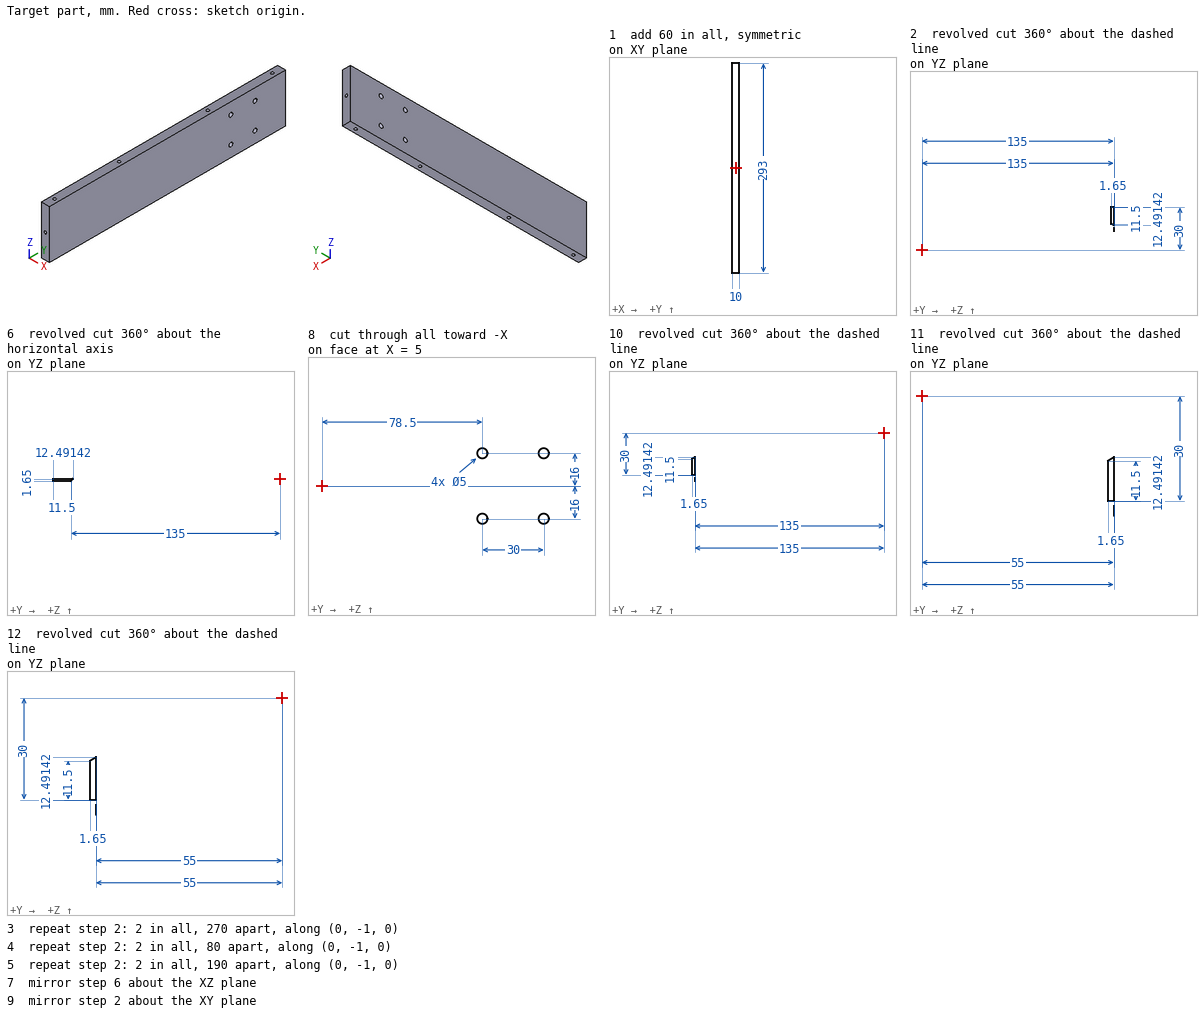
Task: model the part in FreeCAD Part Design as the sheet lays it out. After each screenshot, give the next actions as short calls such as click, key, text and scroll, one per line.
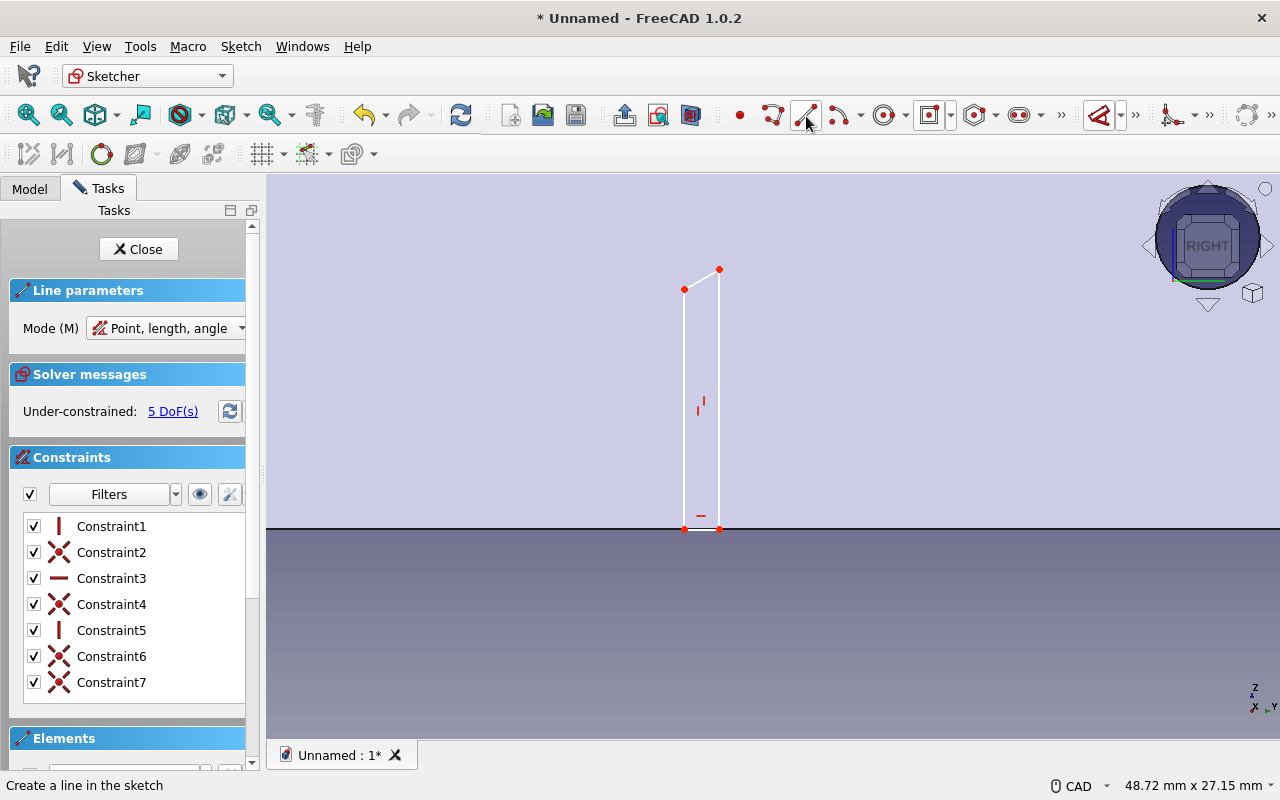
click(719, 555)
click(719, 633)
key(Escape)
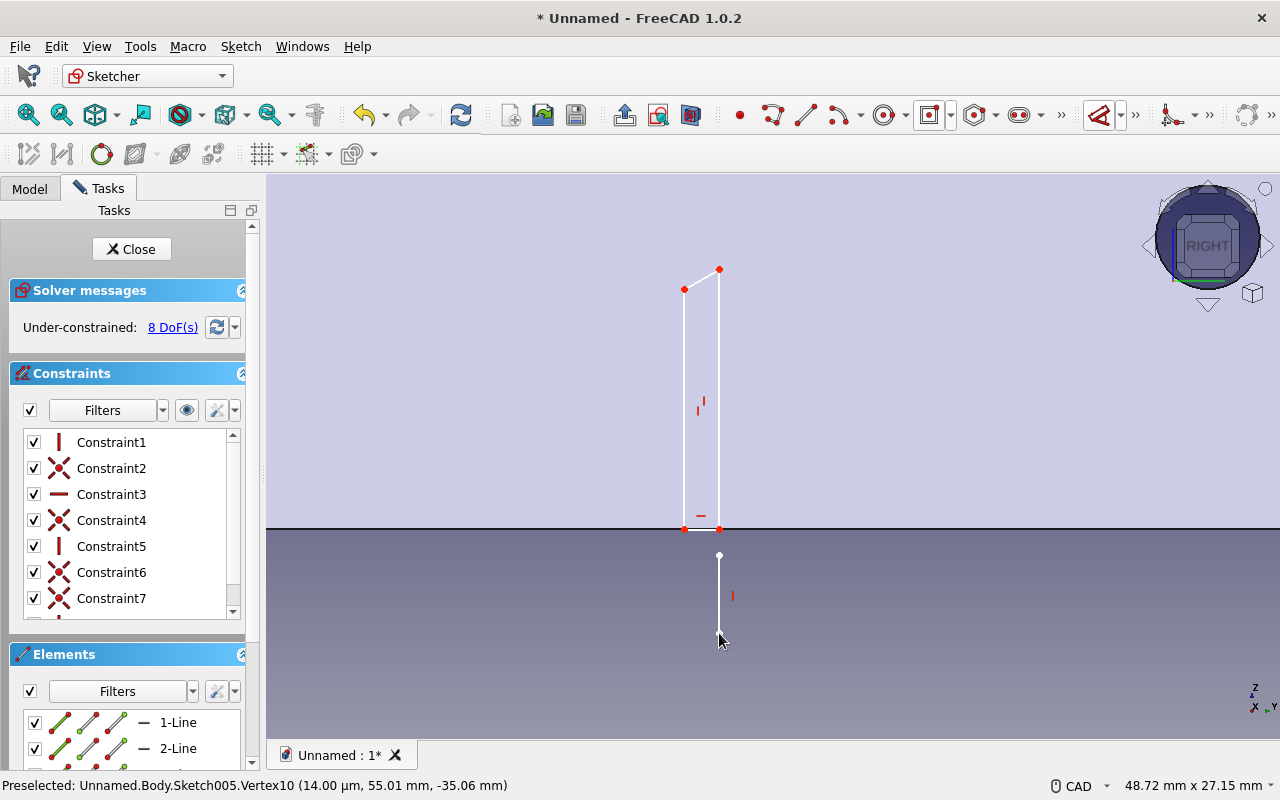
click(719, 579)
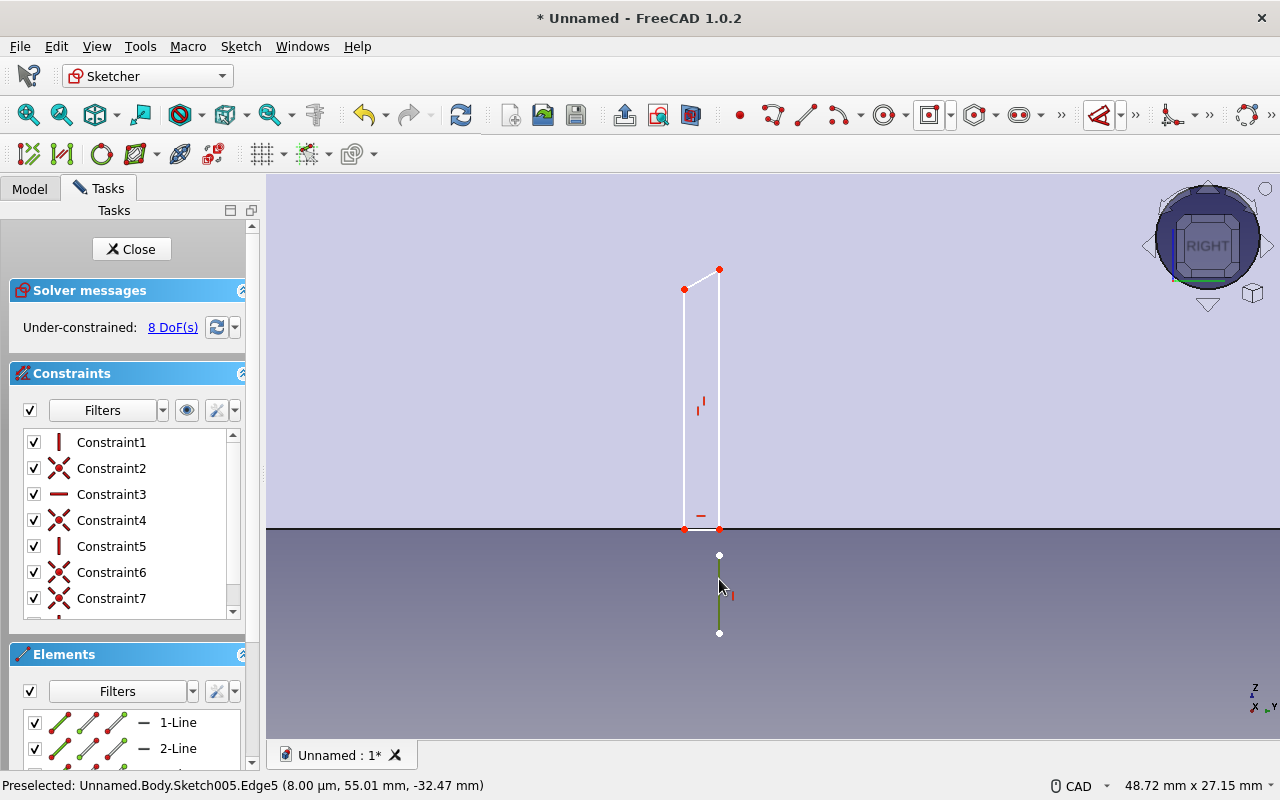
key(g)
key(n)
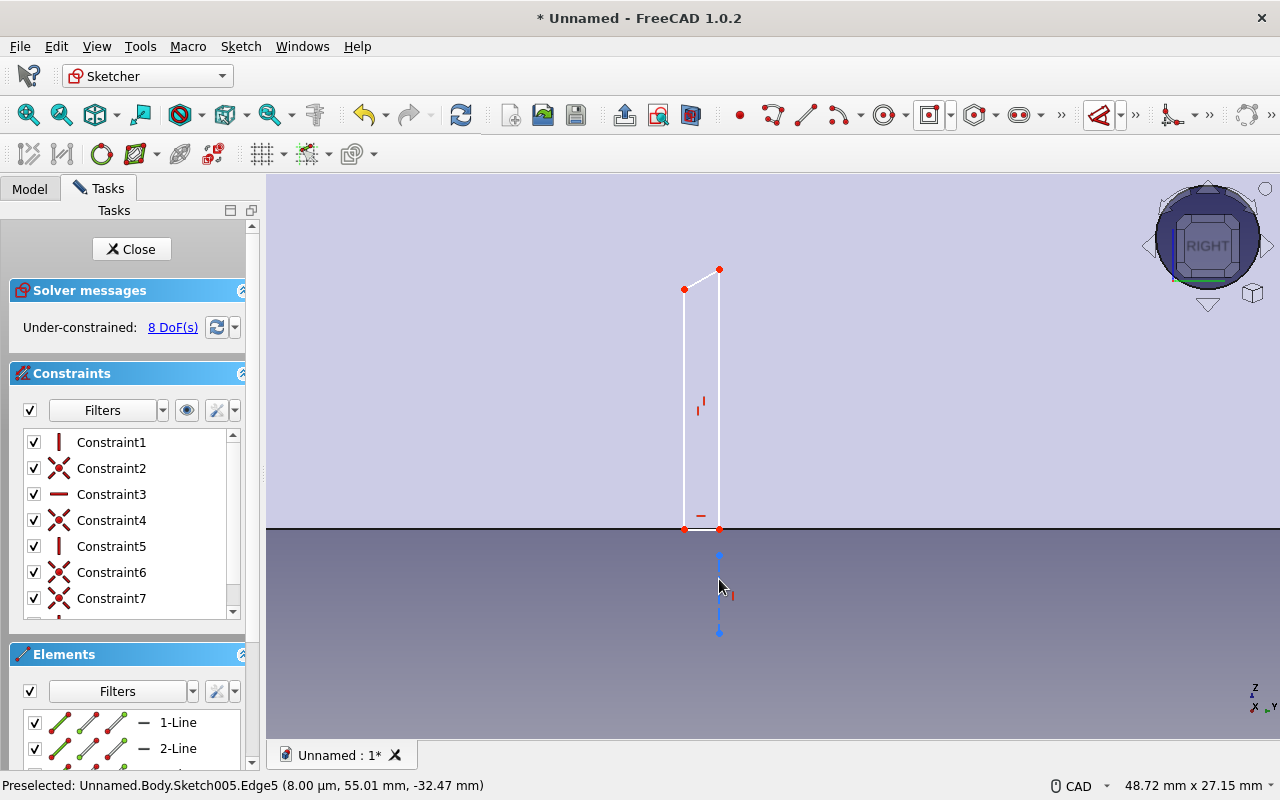
click(684, 530)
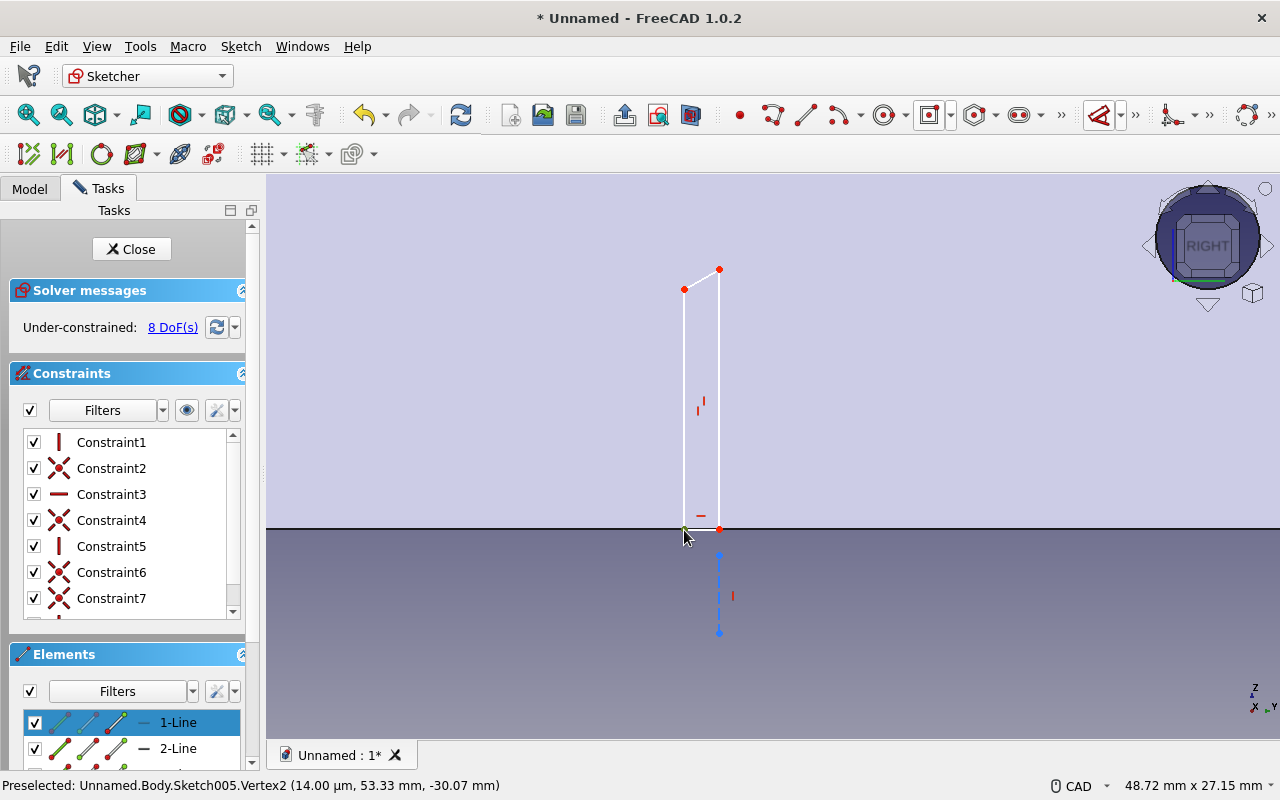
key(i)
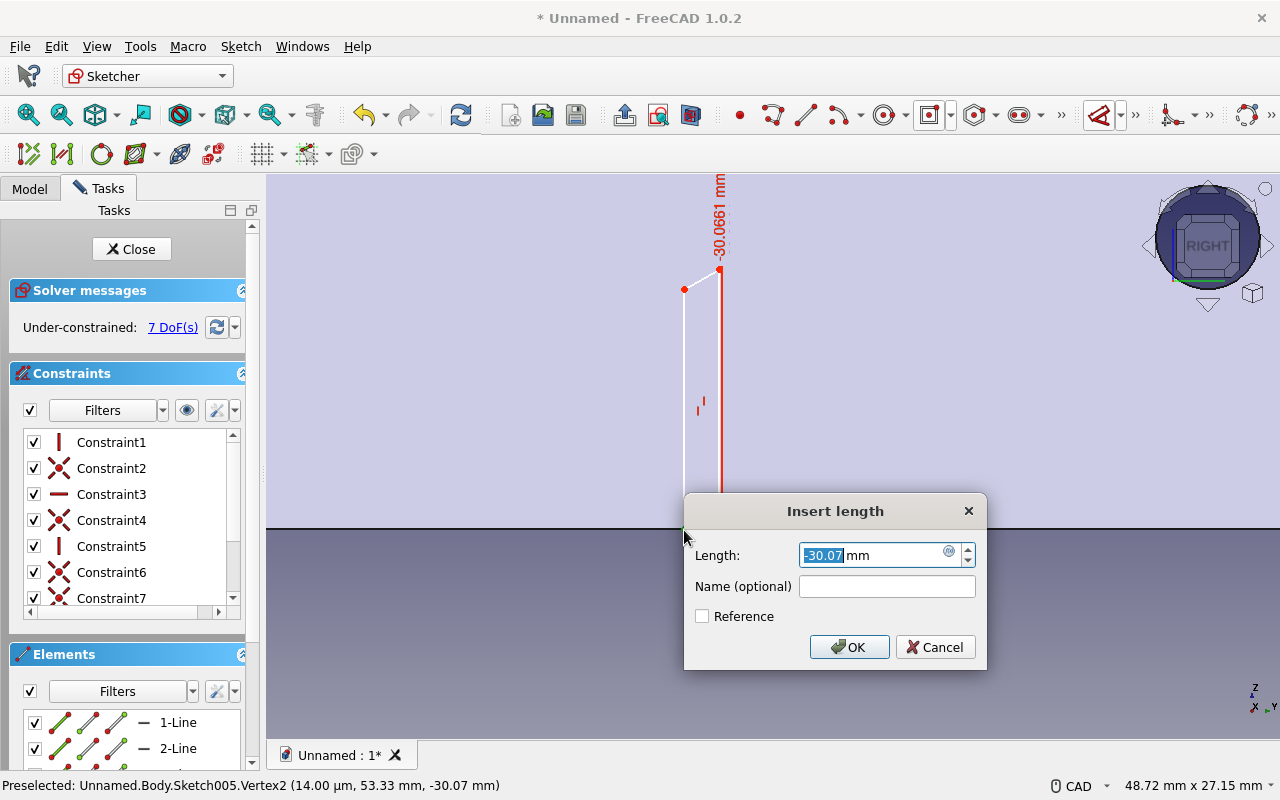
text(-30)
key(Return)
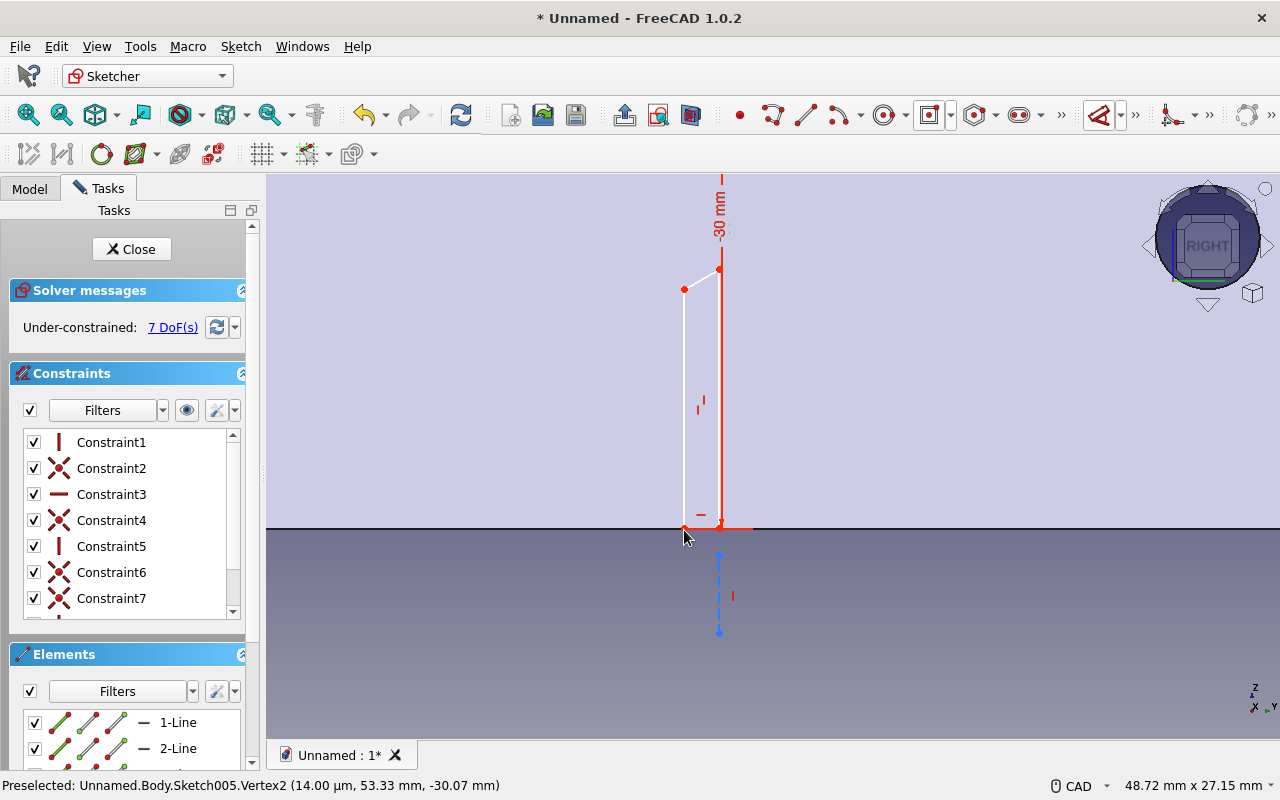
click(719, 529)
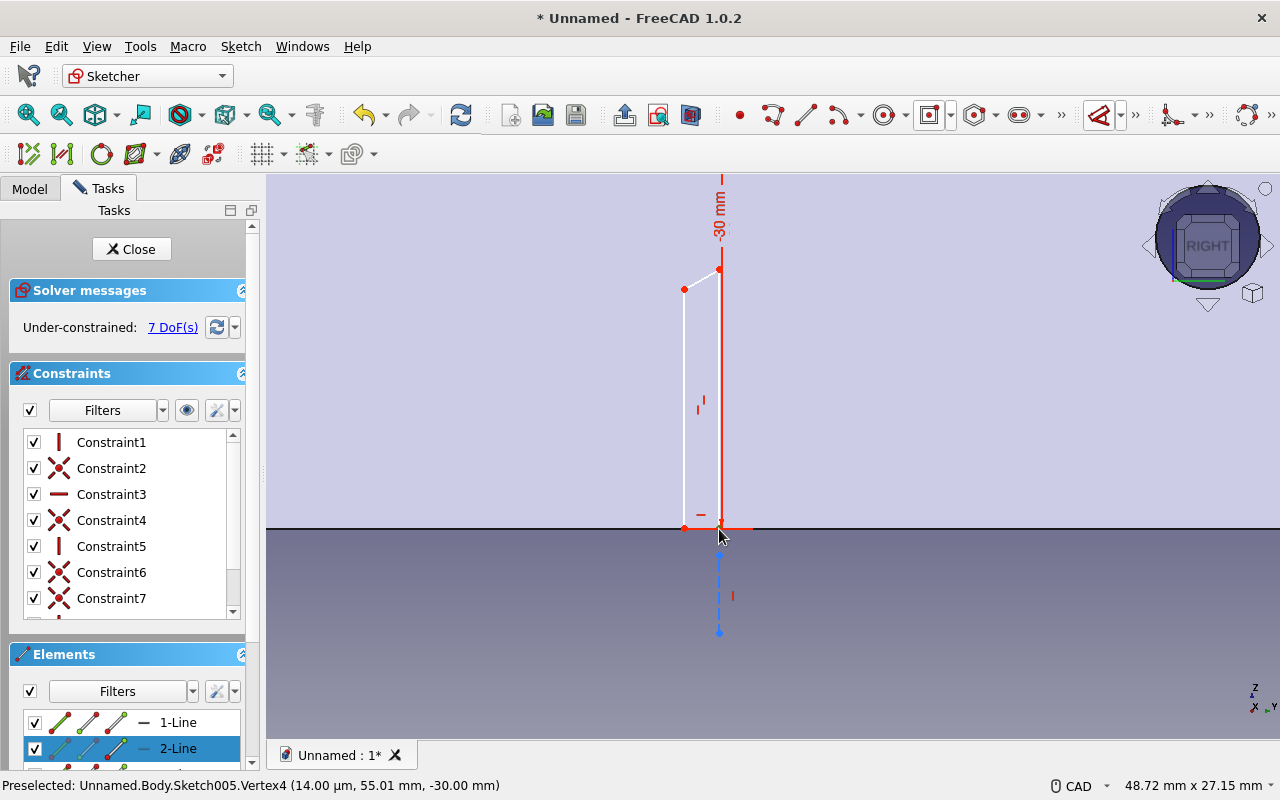
key(l)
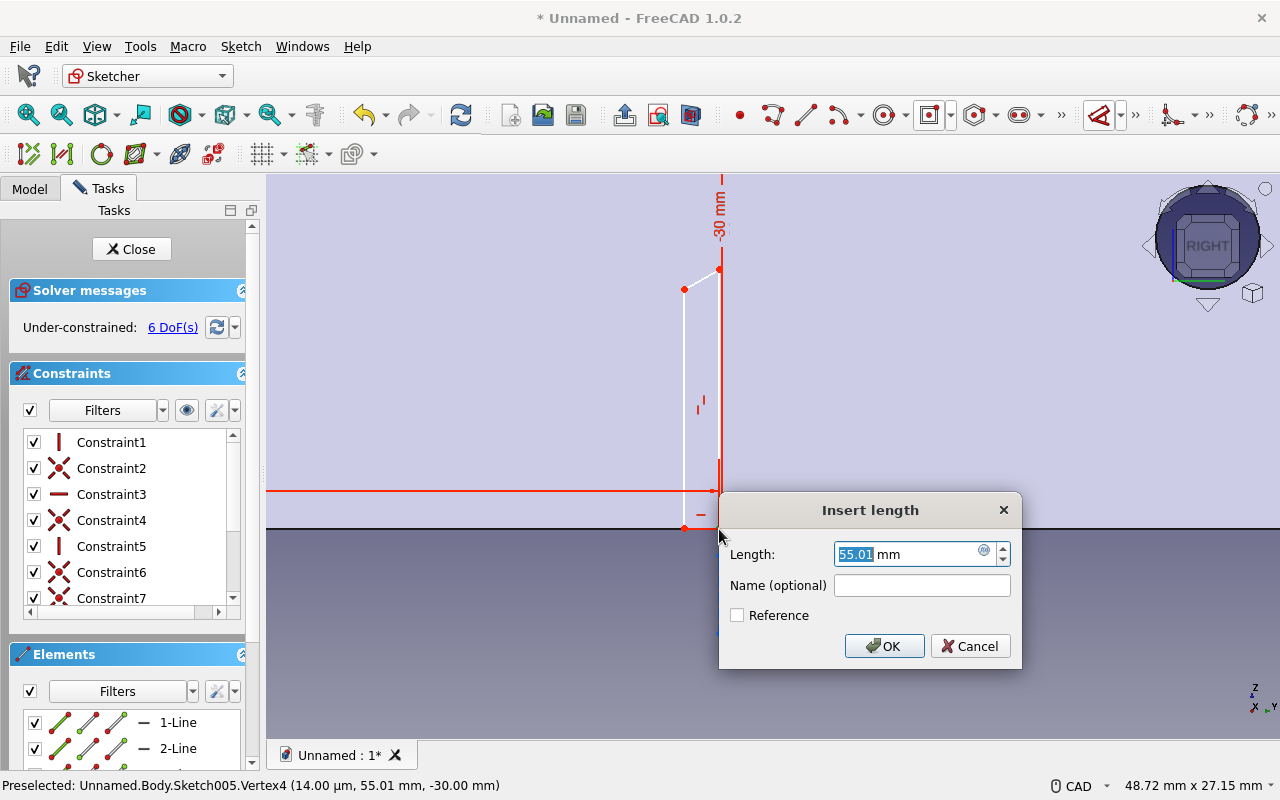
text(55)
key(Return)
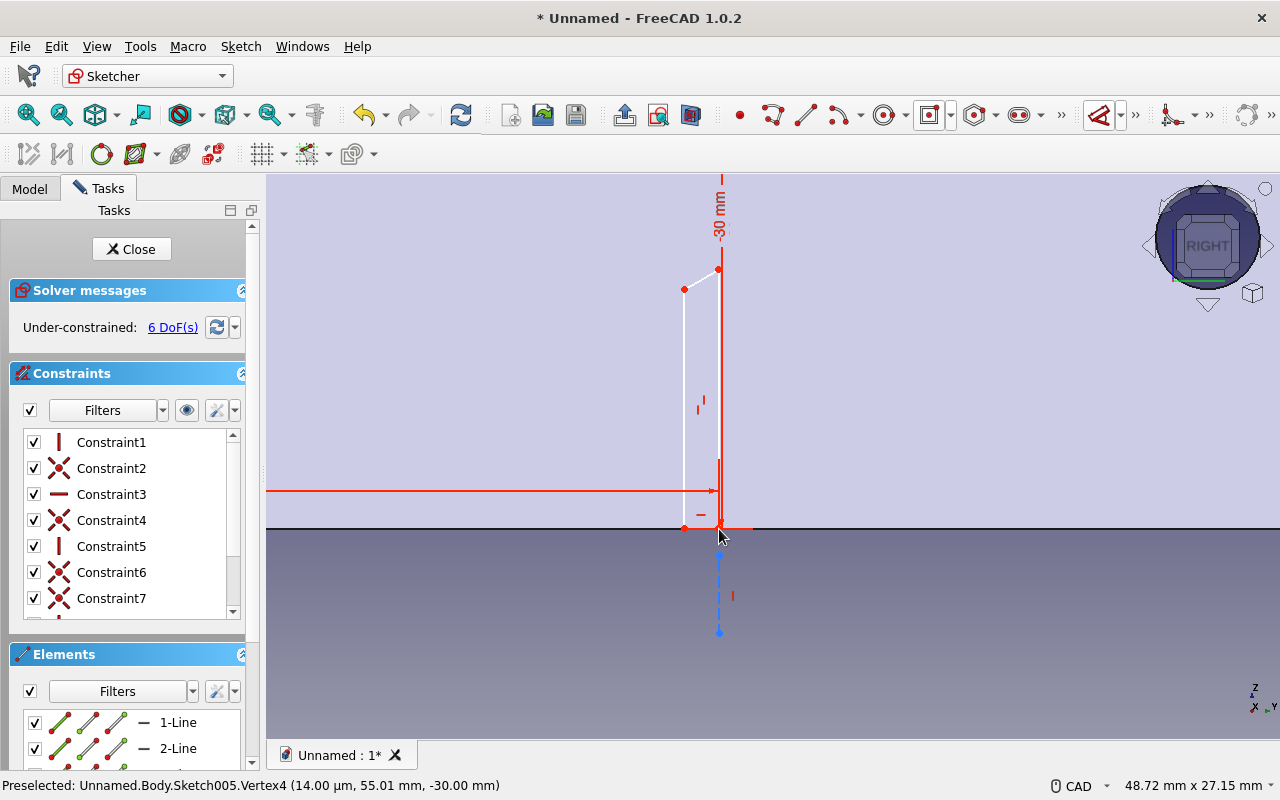
click(719, 556)